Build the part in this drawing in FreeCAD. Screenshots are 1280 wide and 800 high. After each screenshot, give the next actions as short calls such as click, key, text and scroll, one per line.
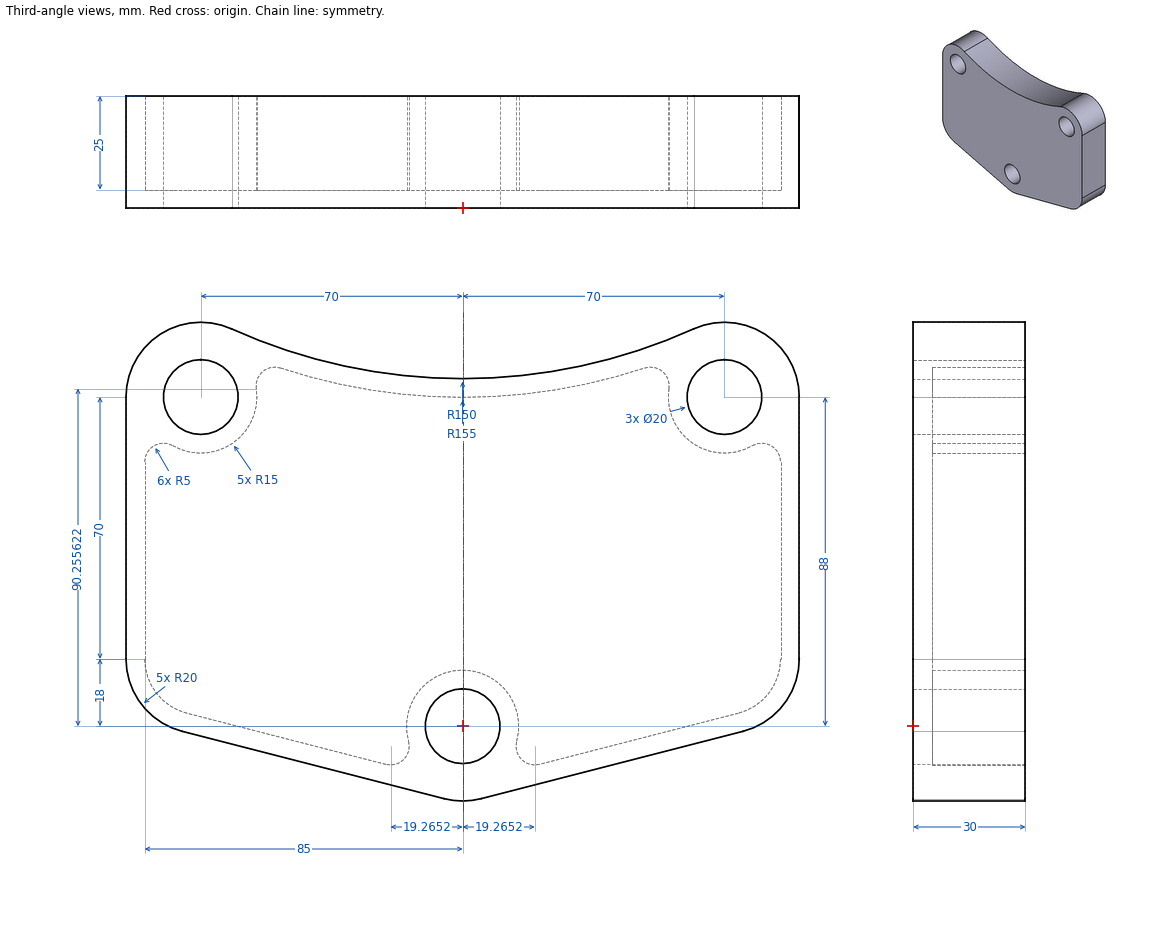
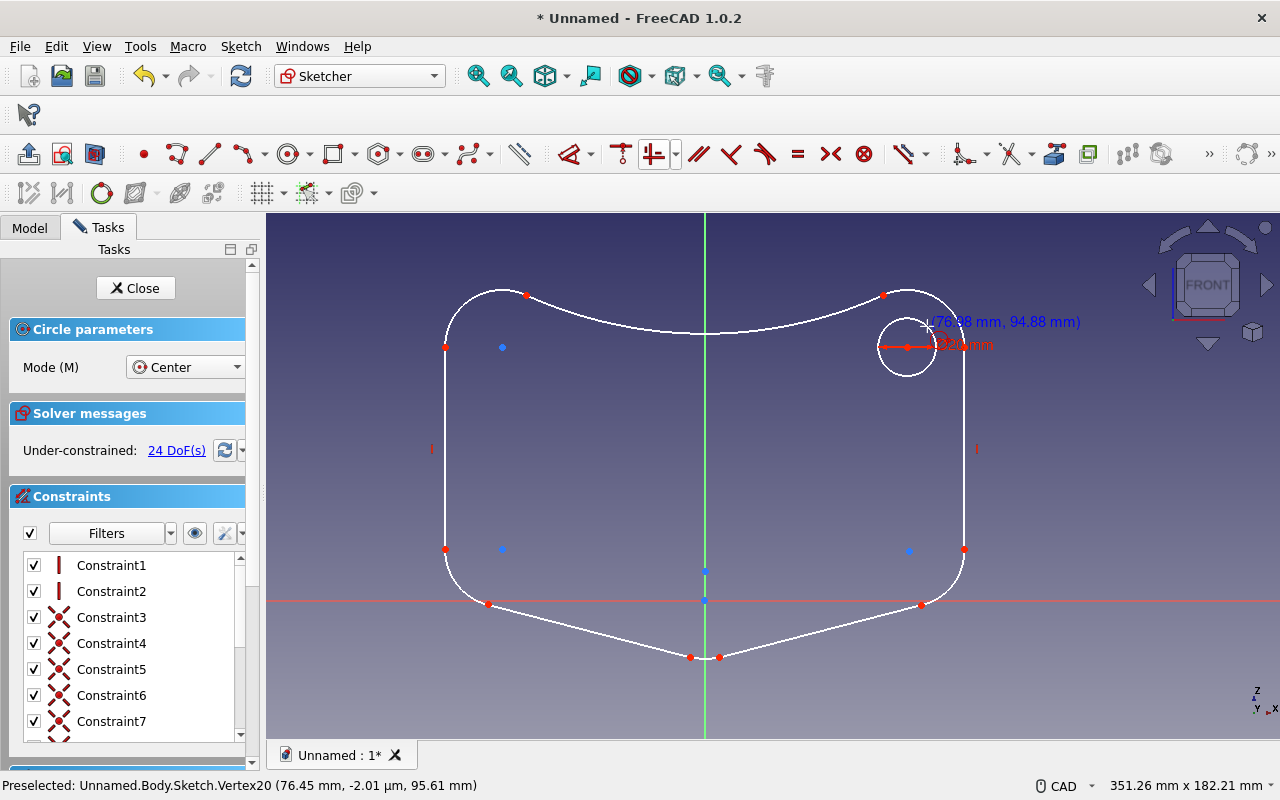
click(503, 347)
move(523, 326)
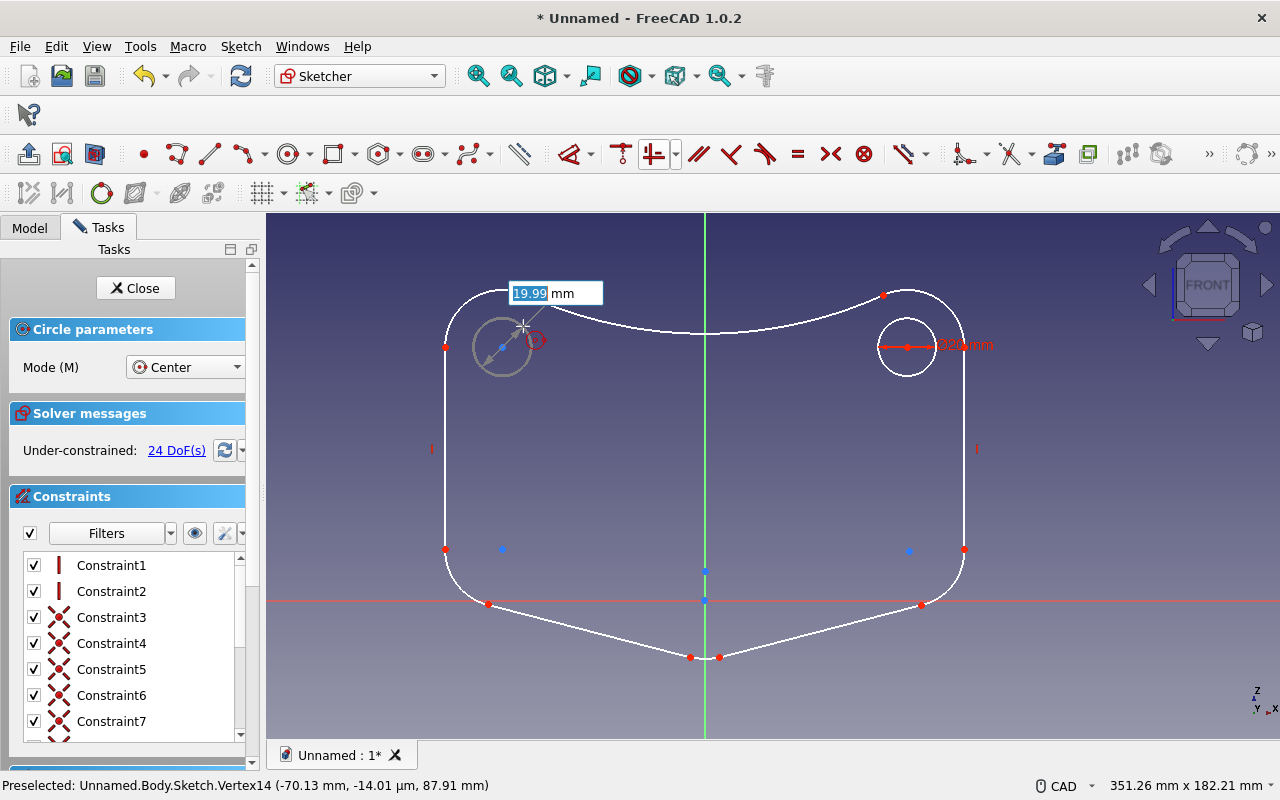
text(20)
key(Return)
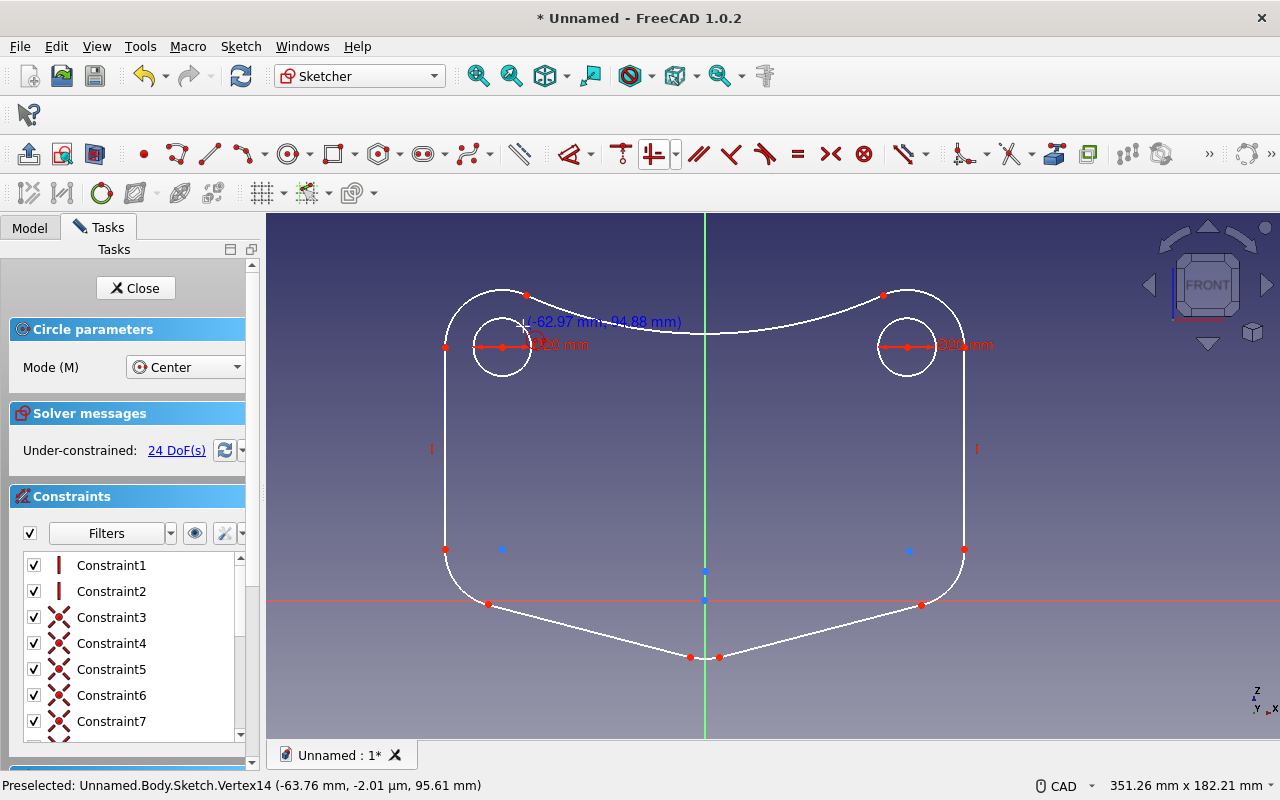
click(705, 601)
move(725, 580)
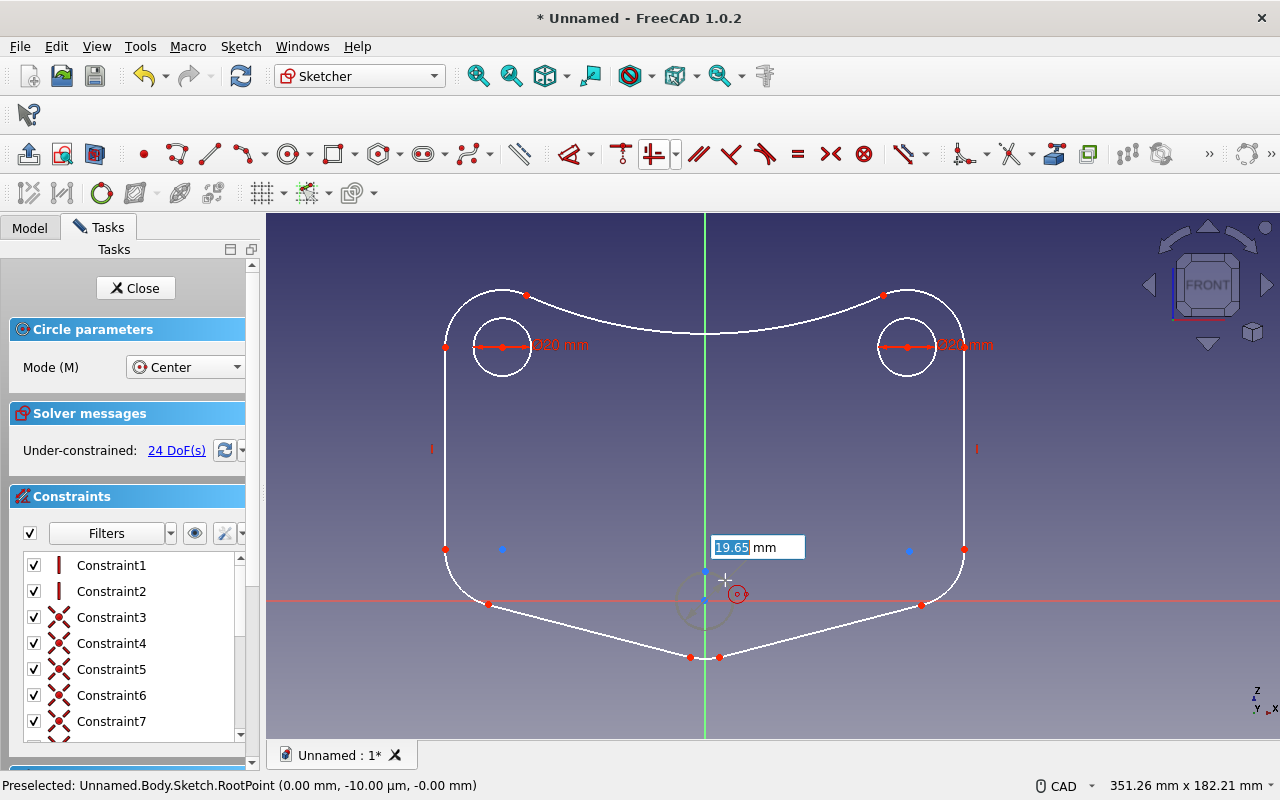
text(20)
key(Return)
key(Escape)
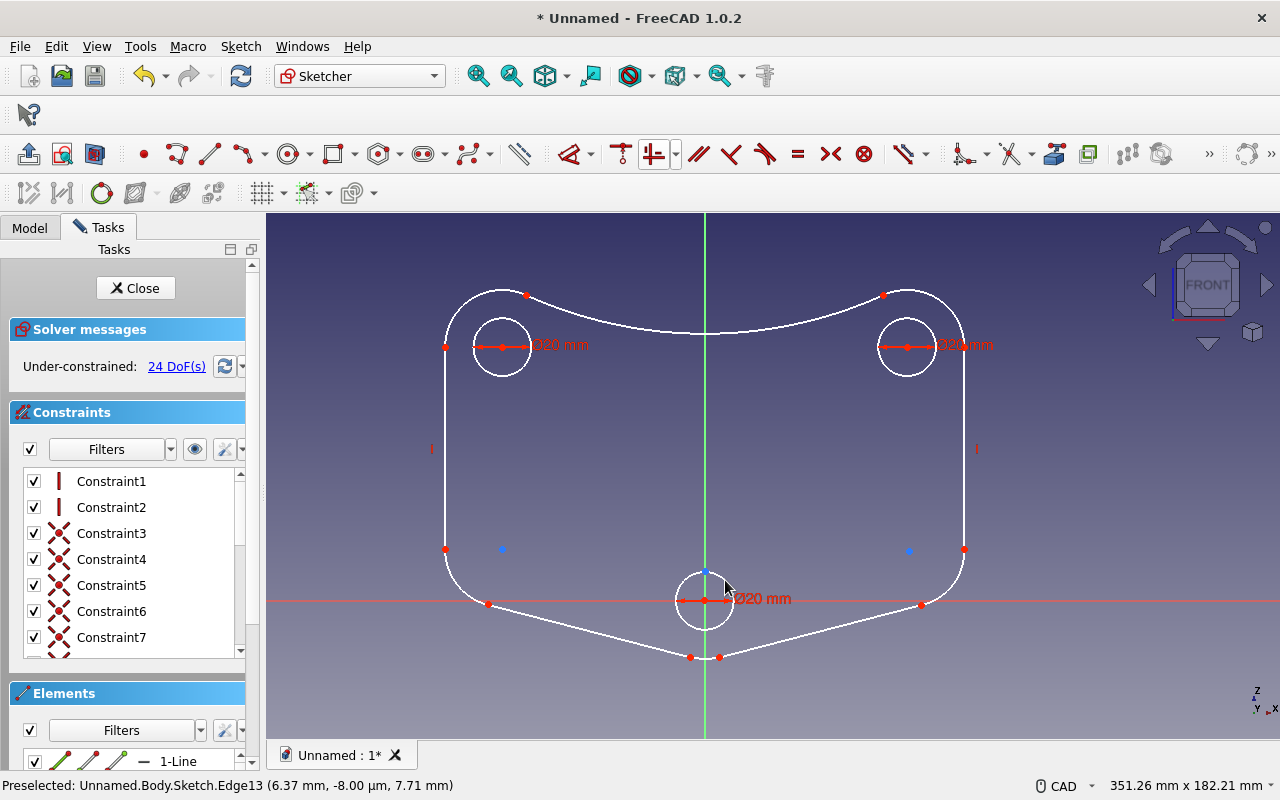
click(630, 642)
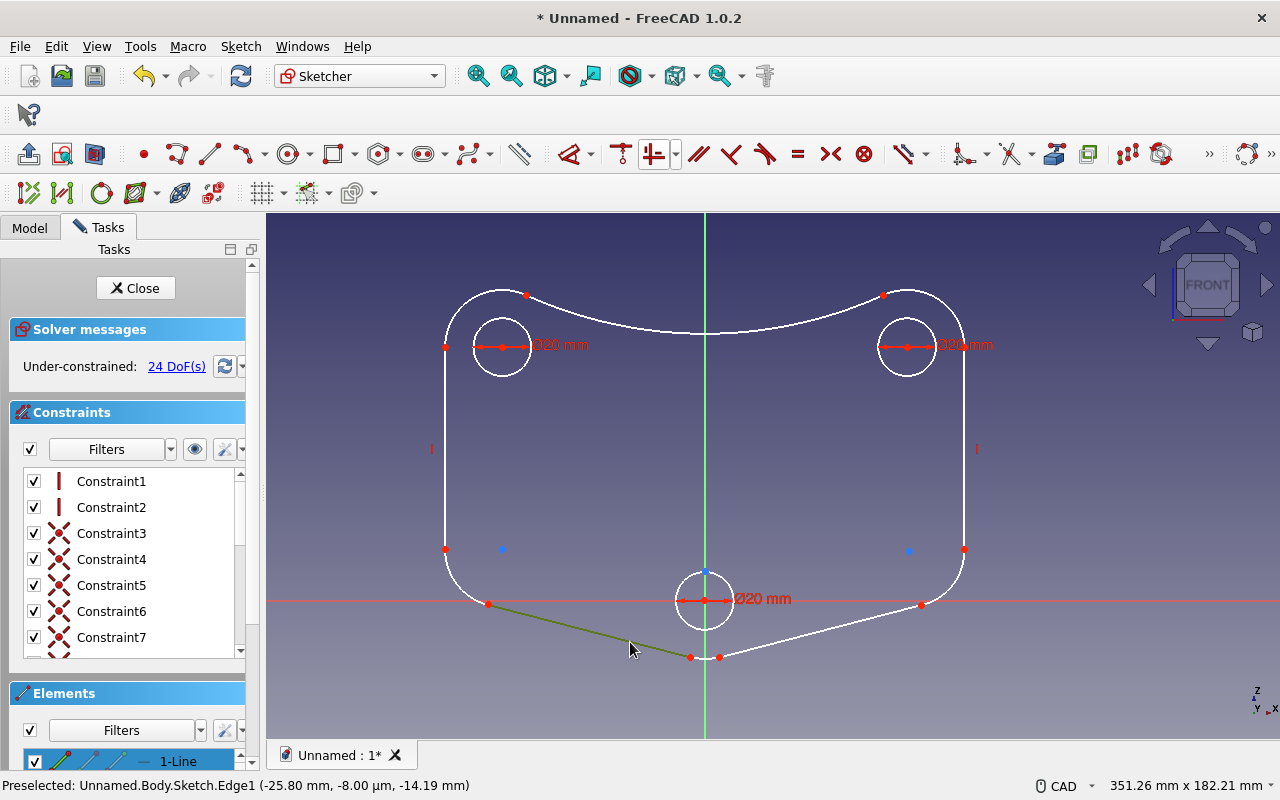
click(450, 572)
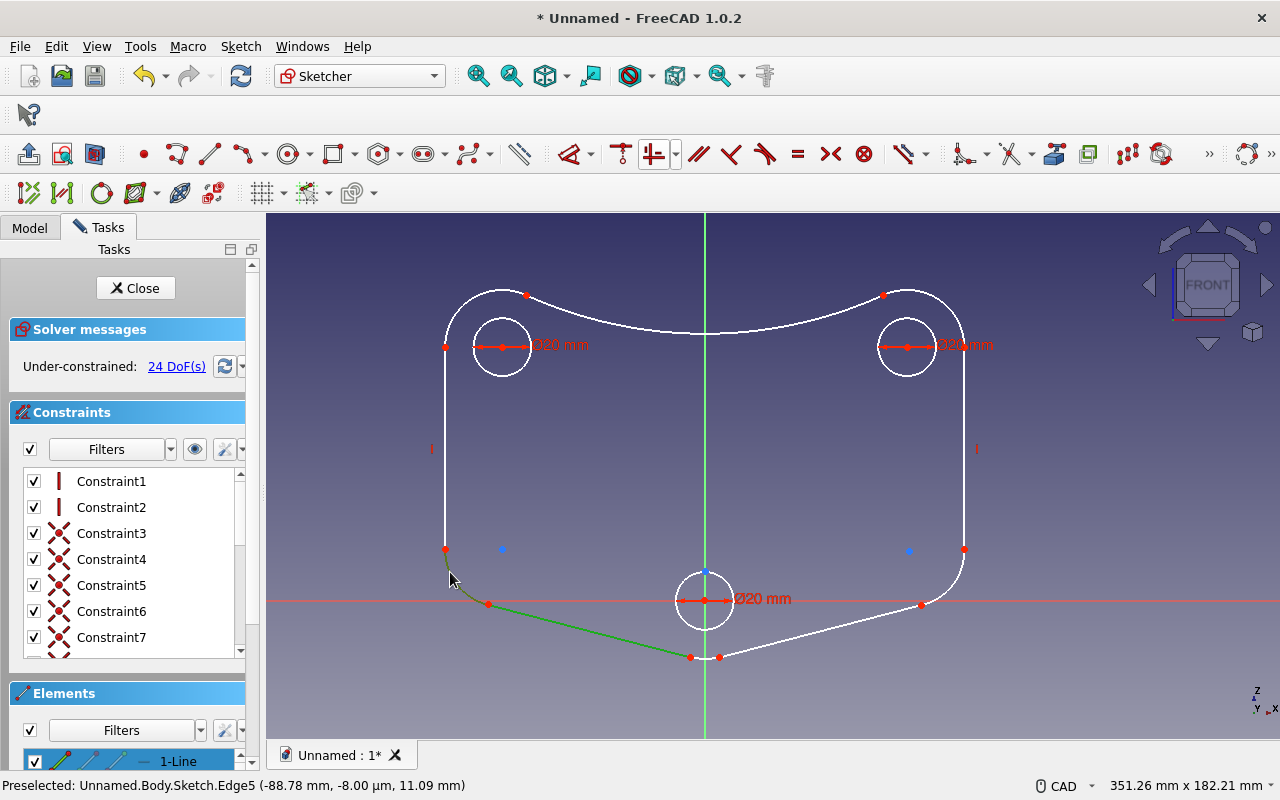
click(765, 154)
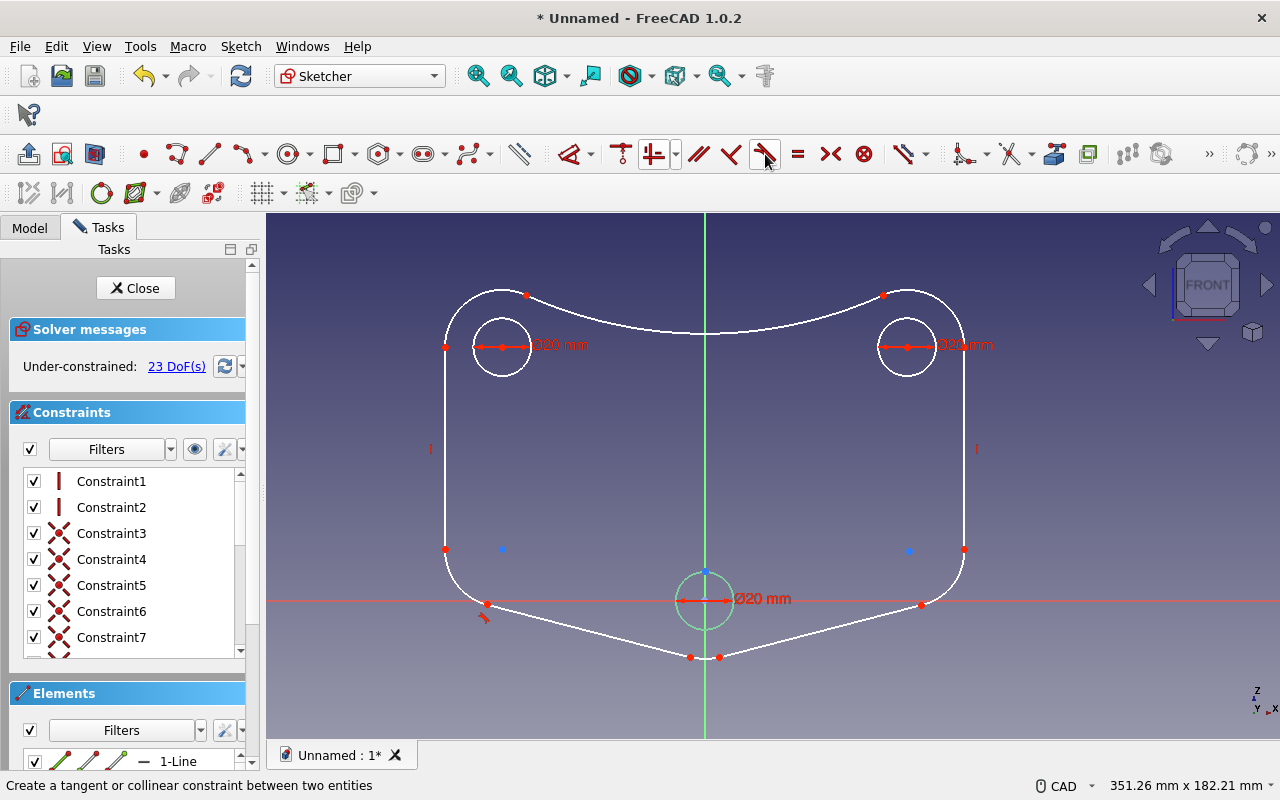
click(629, 642)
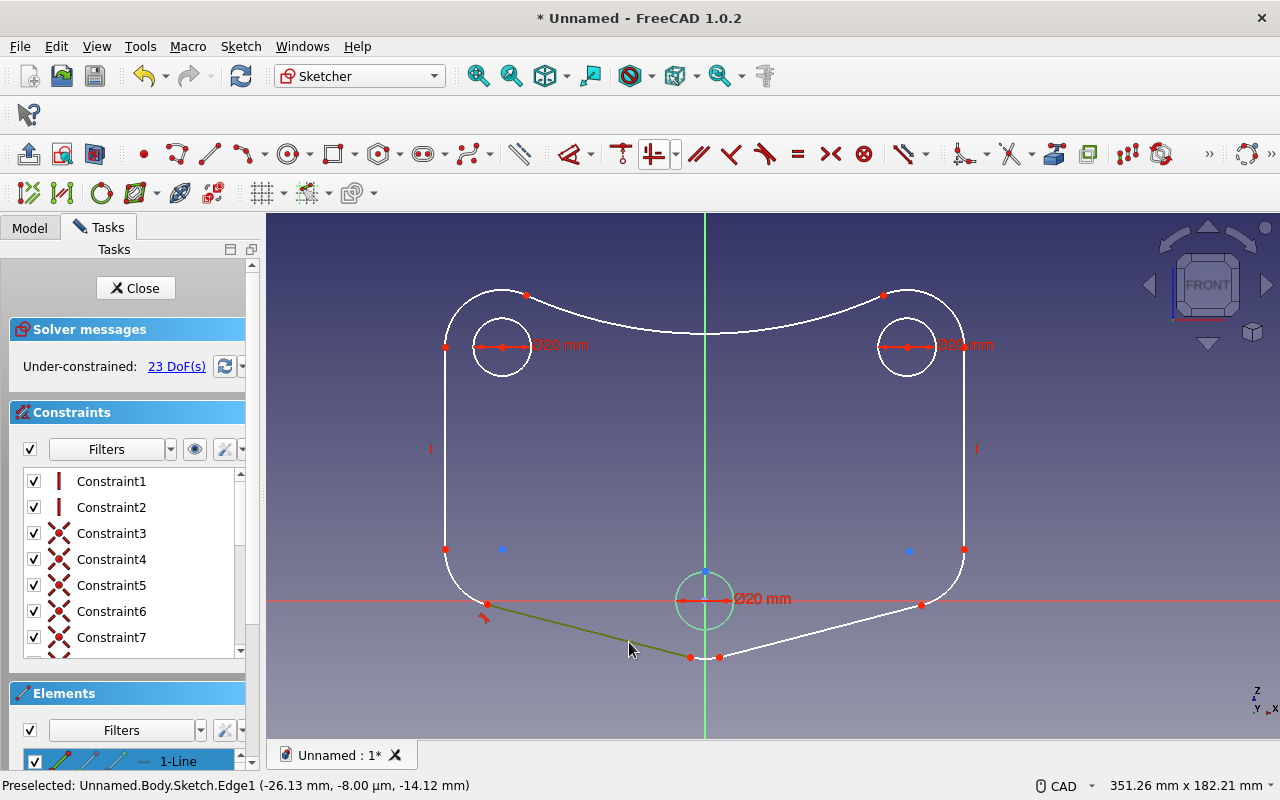
click(705, 659)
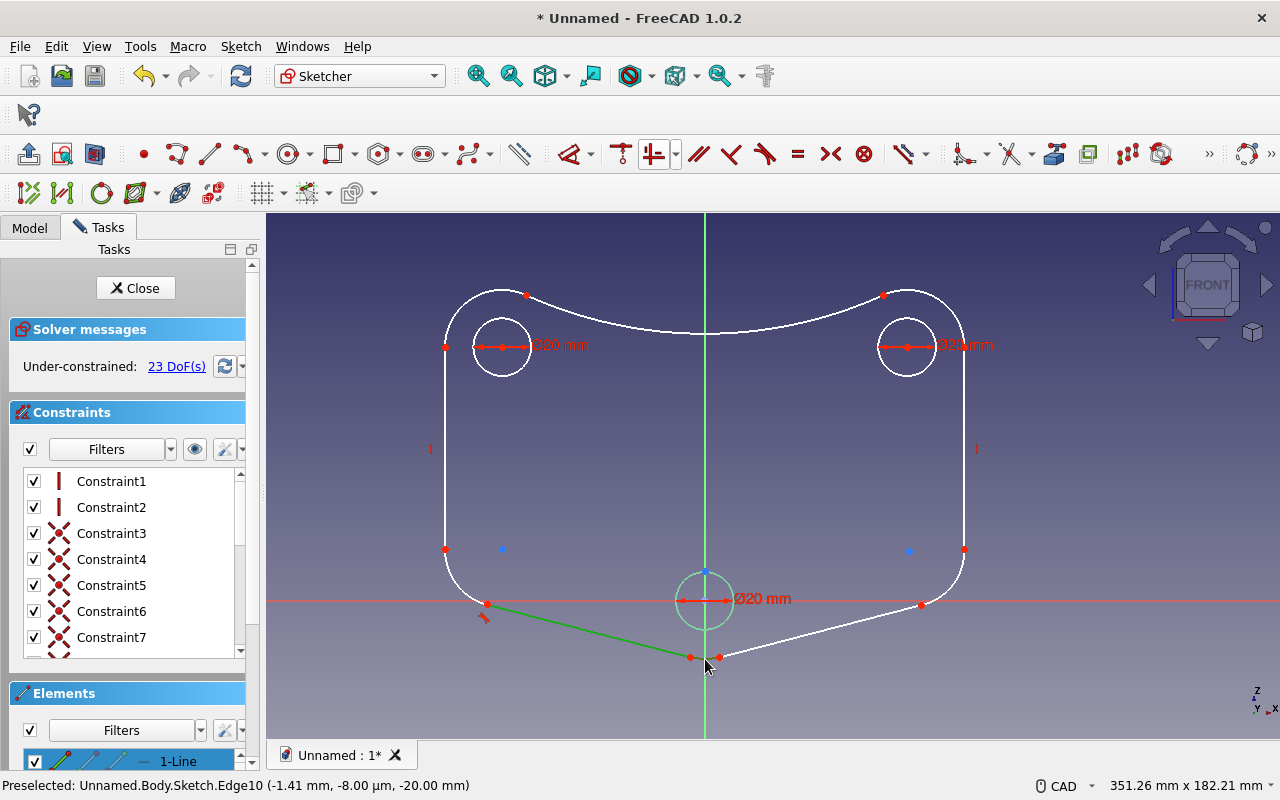
click(765, 154)